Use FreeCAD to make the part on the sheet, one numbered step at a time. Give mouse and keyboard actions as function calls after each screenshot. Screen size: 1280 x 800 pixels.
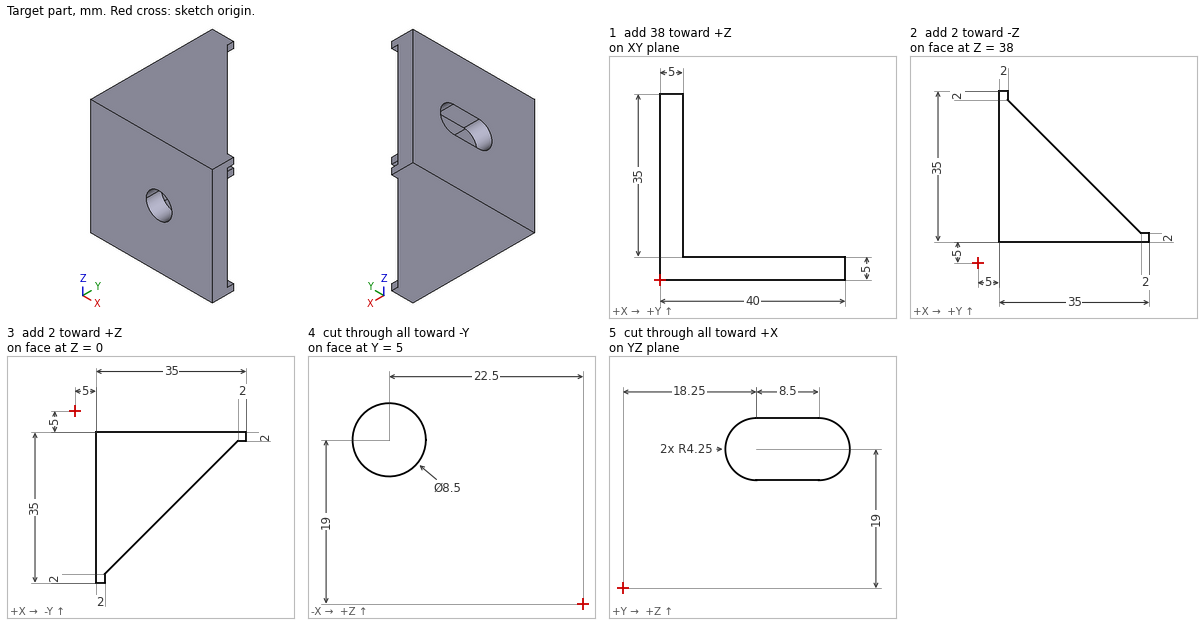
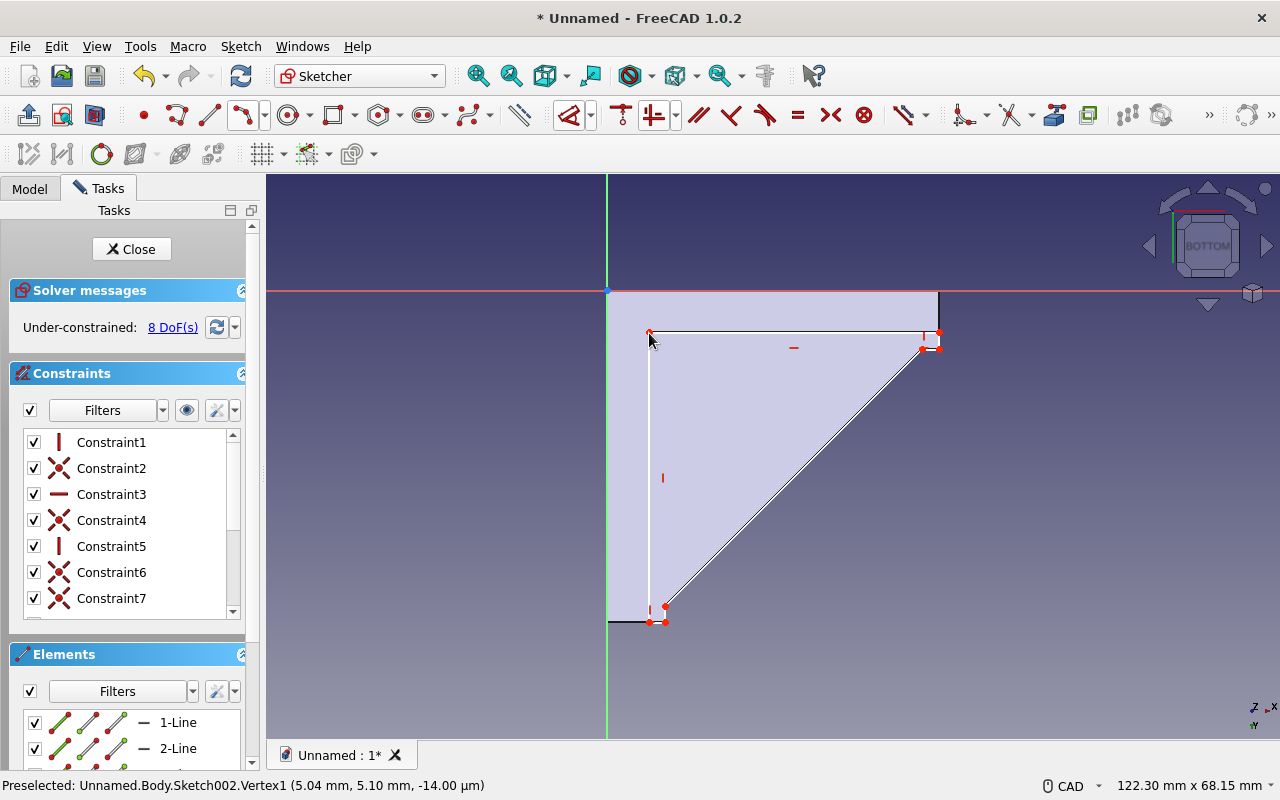
scroll(657, 623, up, 5)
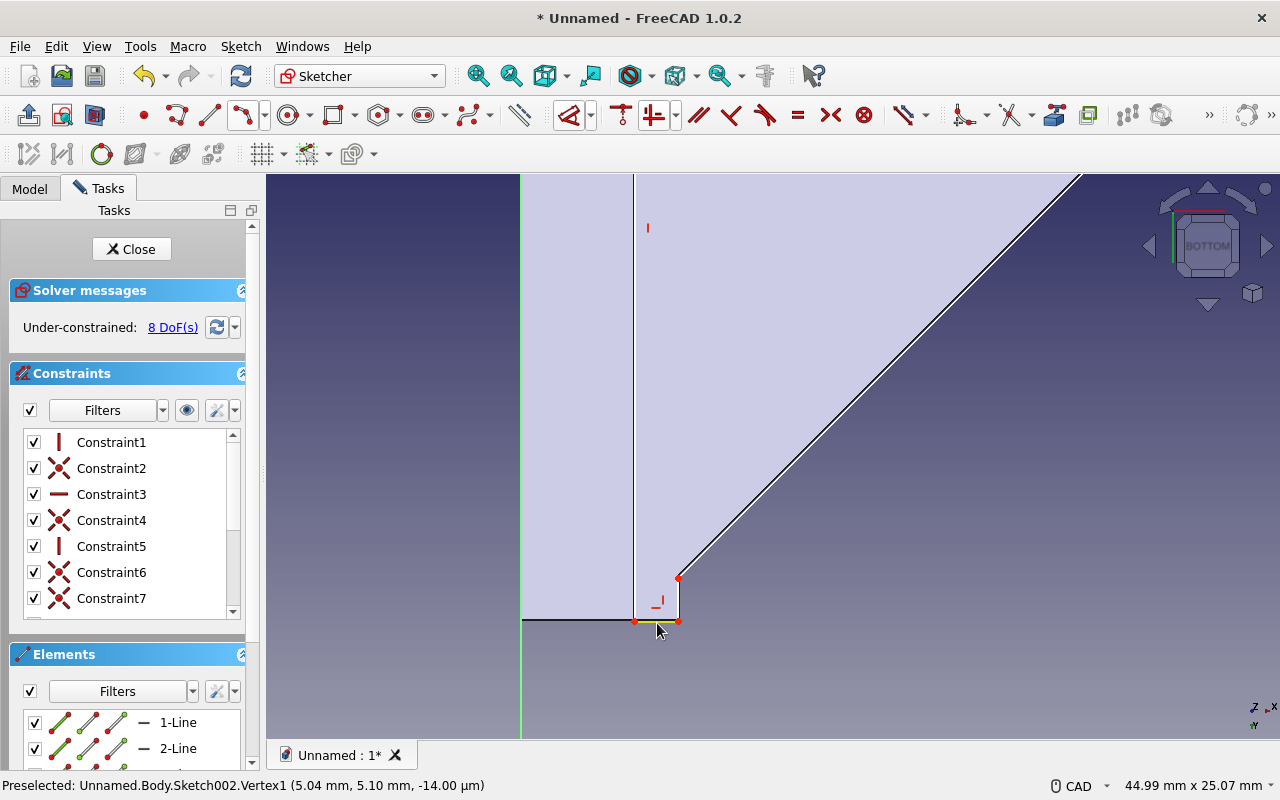
click(656, 622)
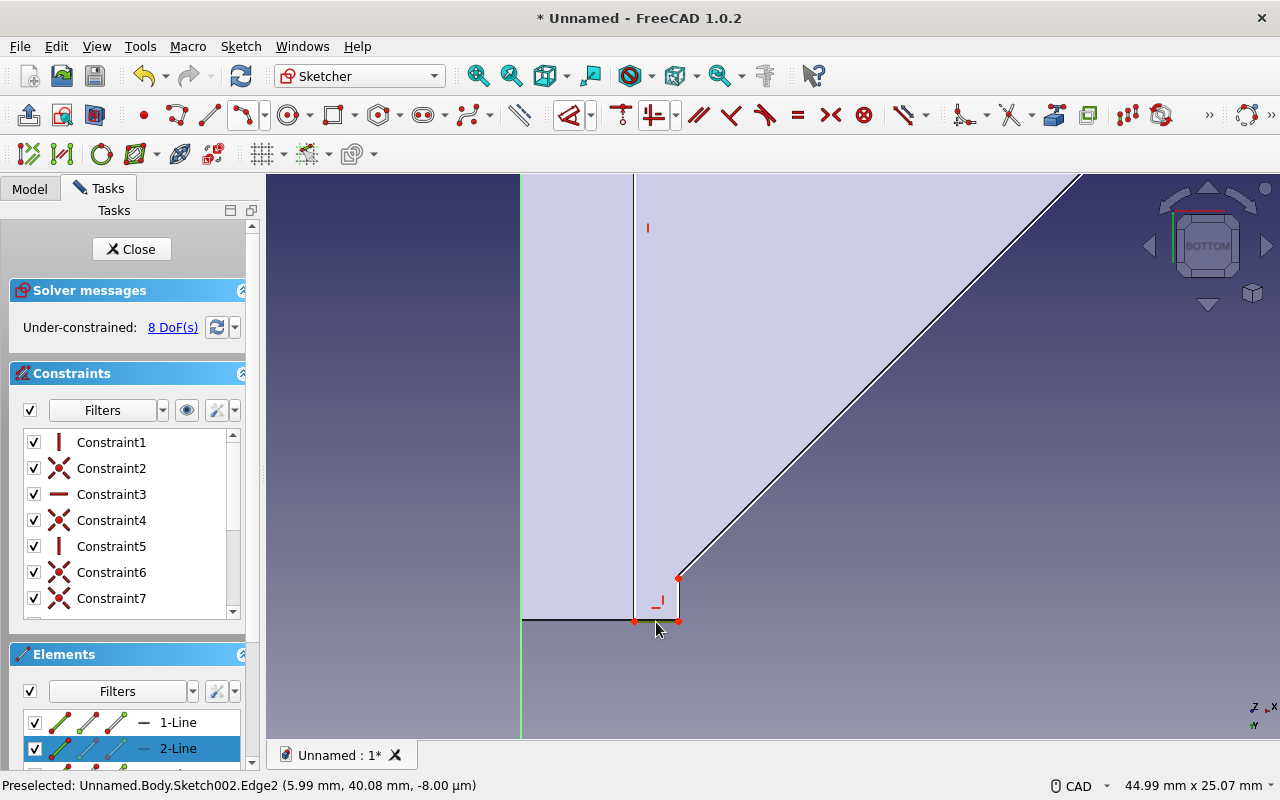
click(590, 116)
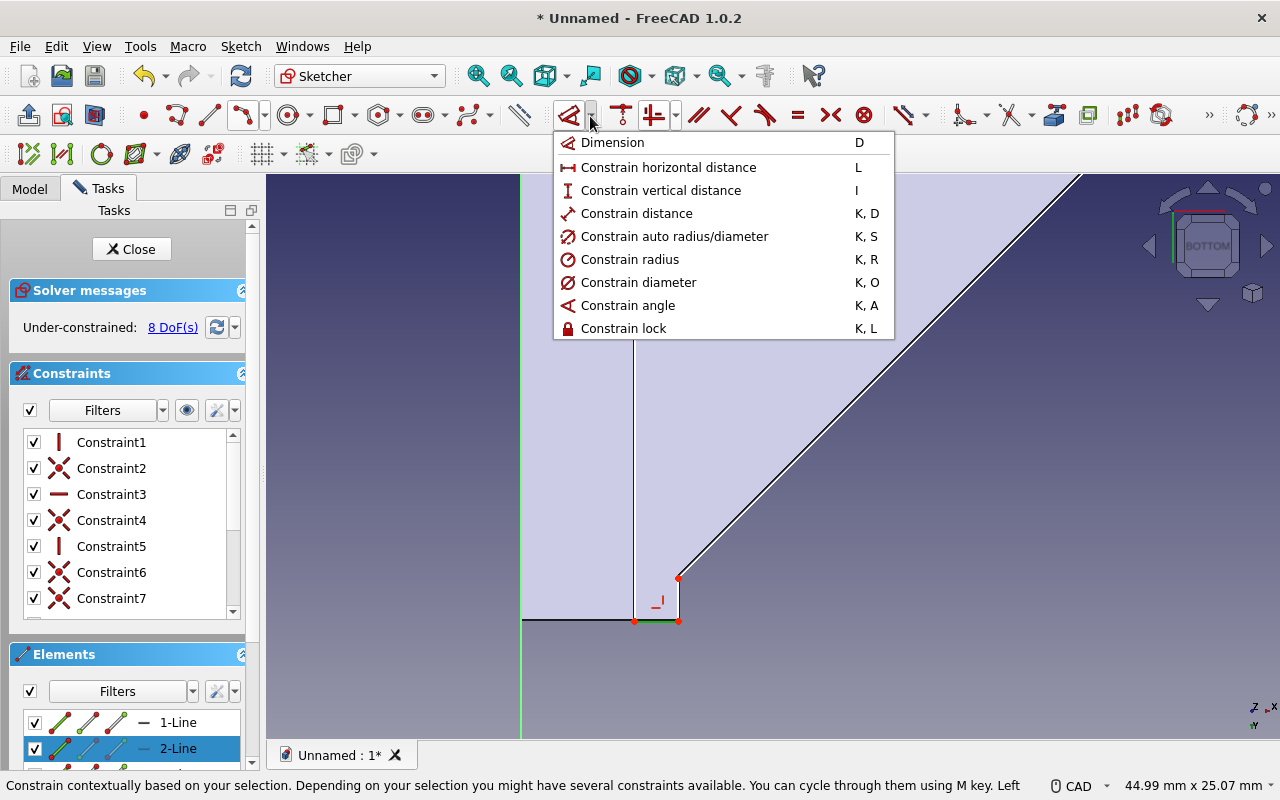
click(724, 168)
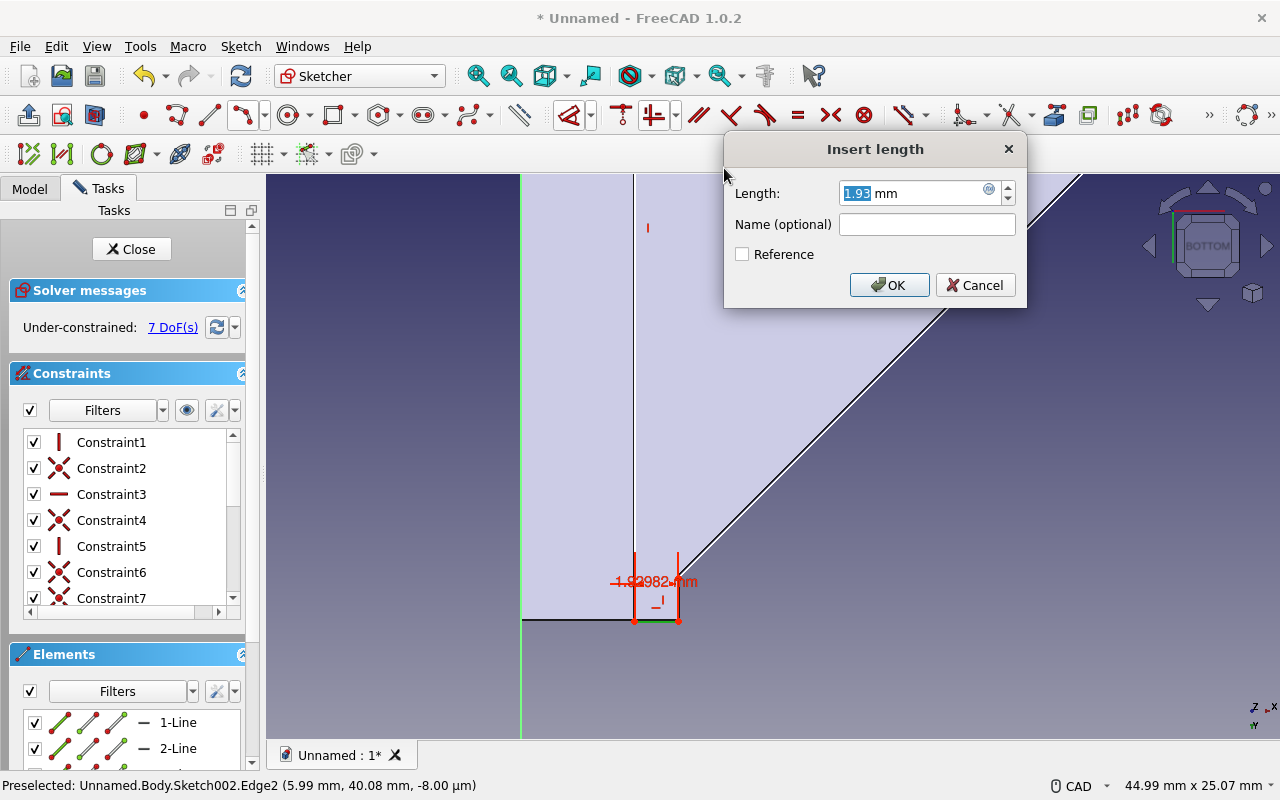
text(2)
key(Return)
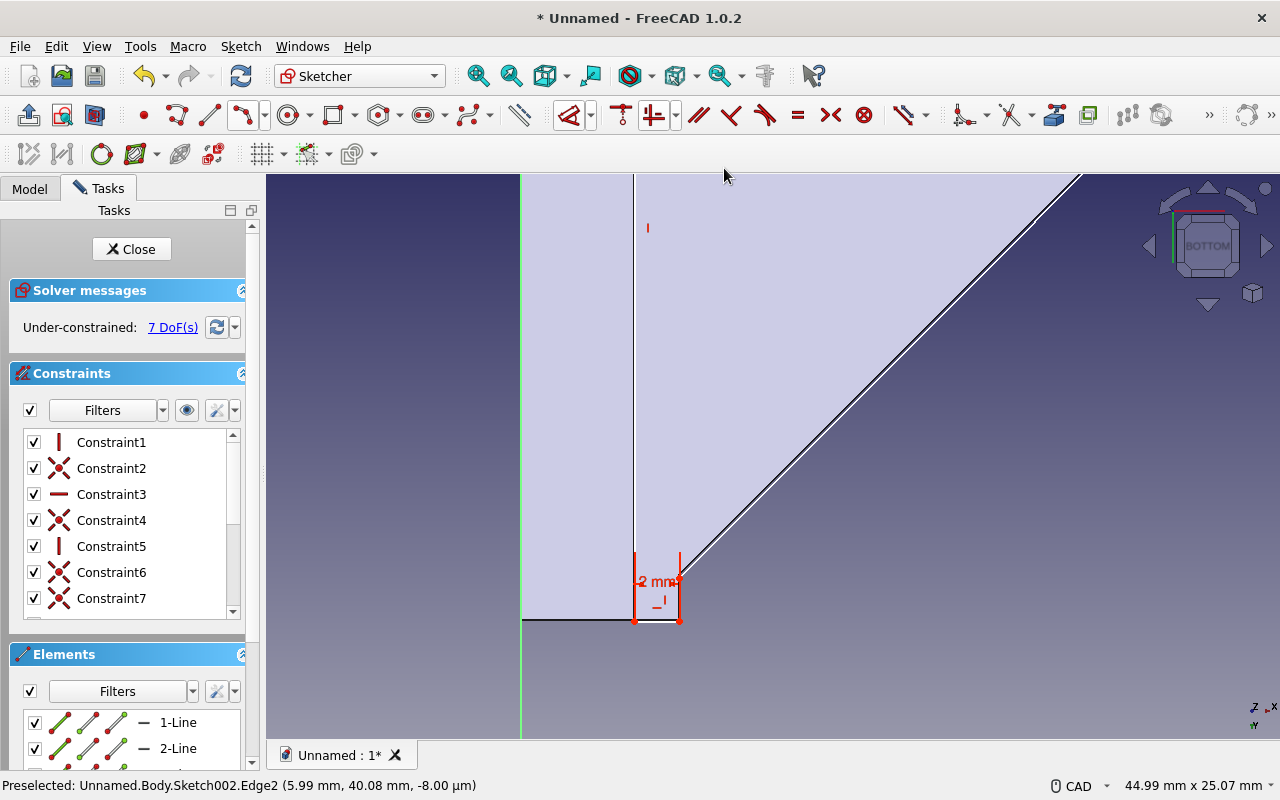
click(680, 609)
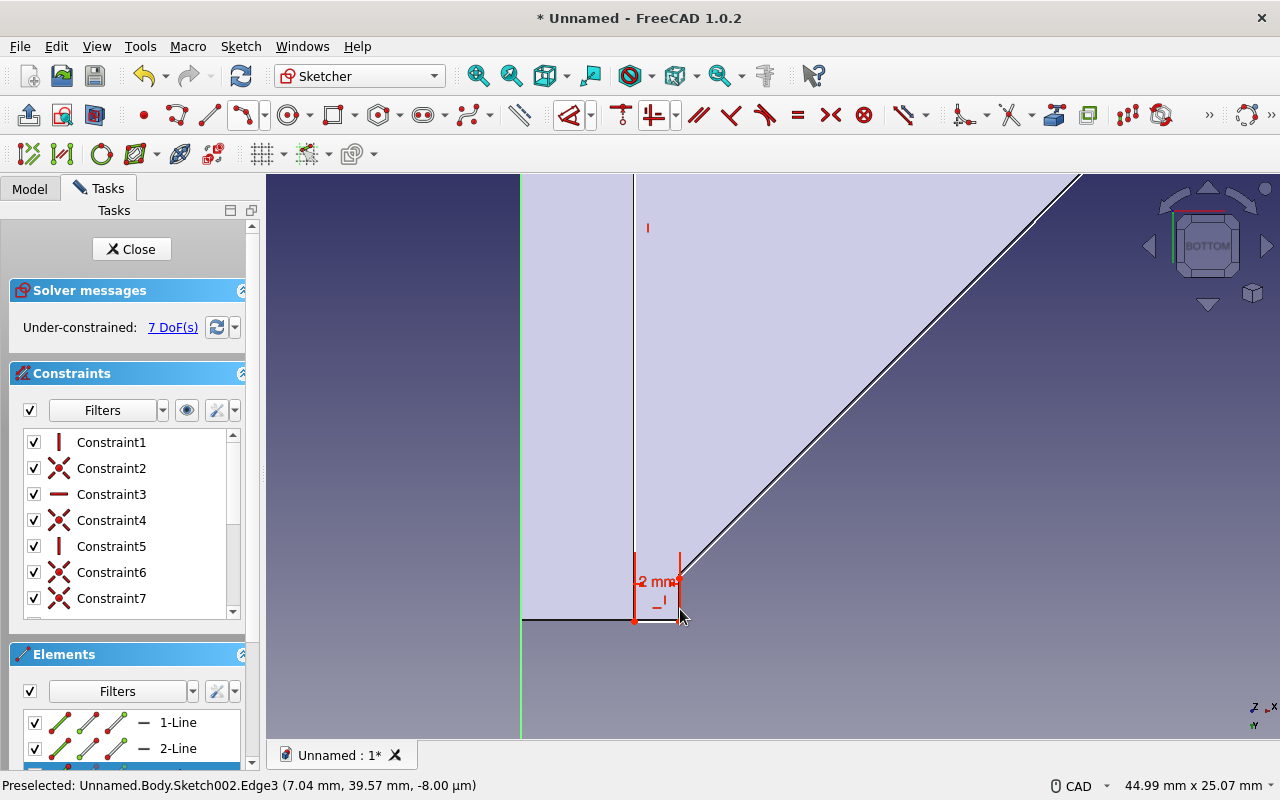
click(590, 116)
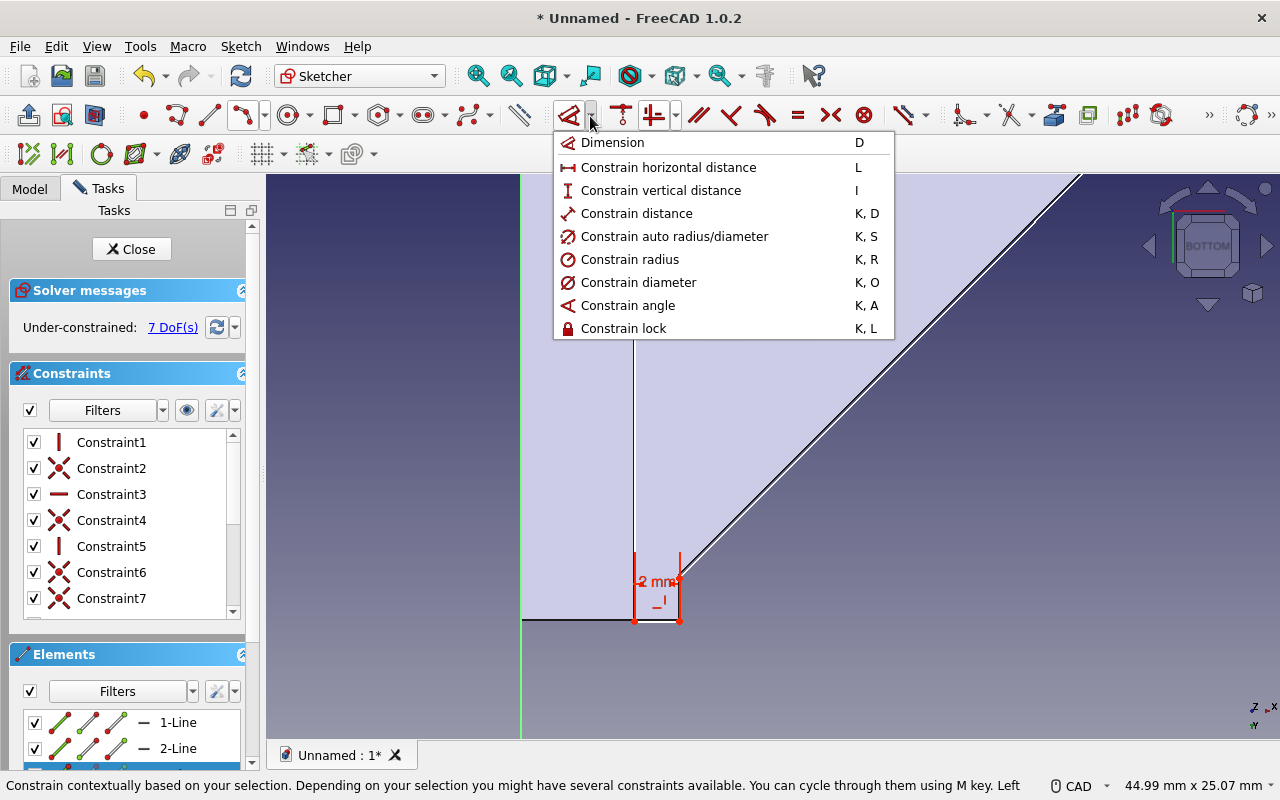
click(724, 190)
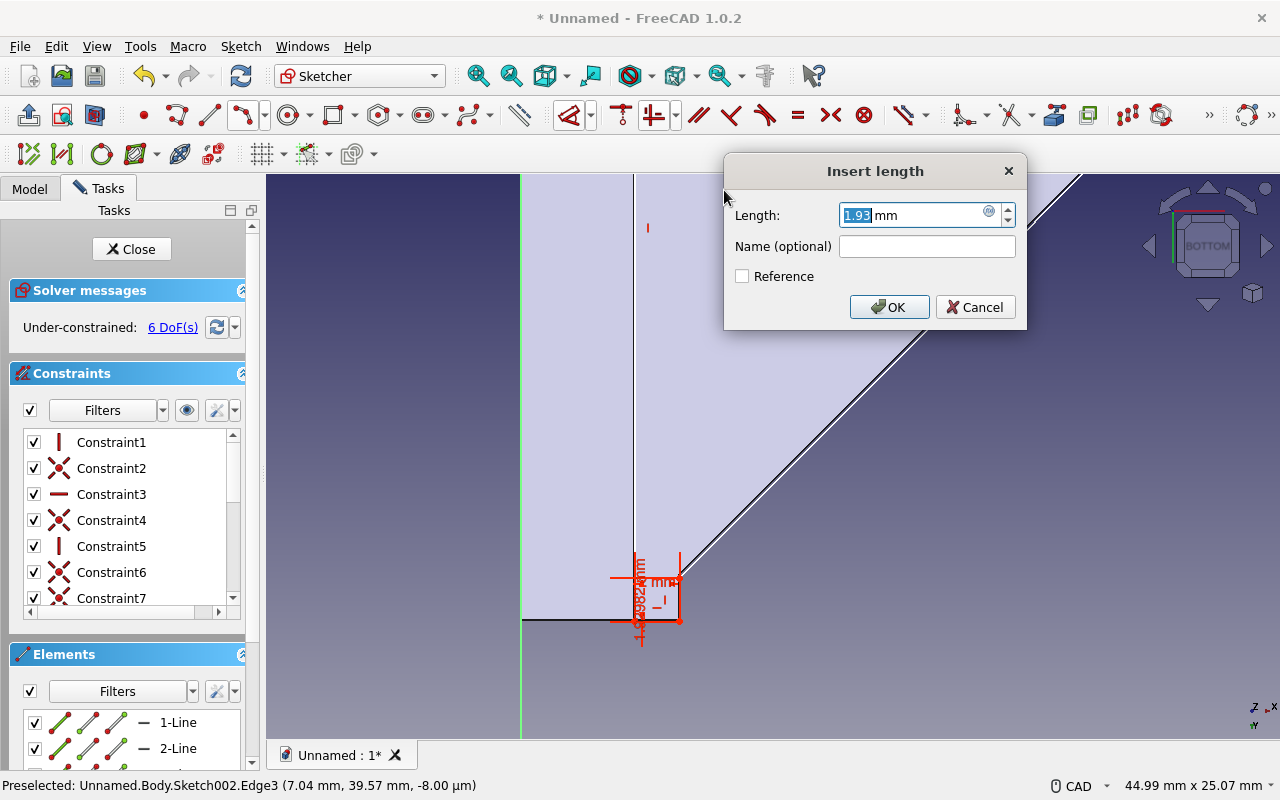
text(2)
key(Return)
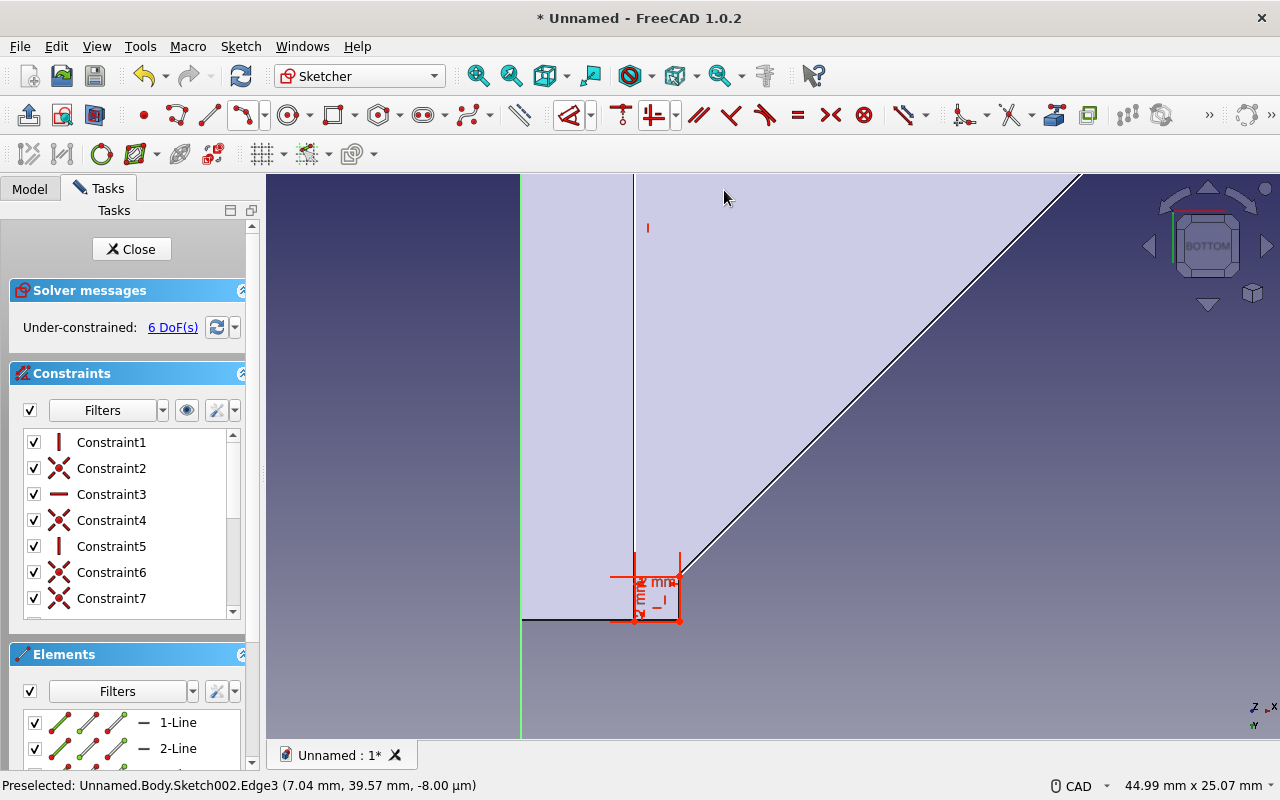
scroll(549, 624, down, 5)